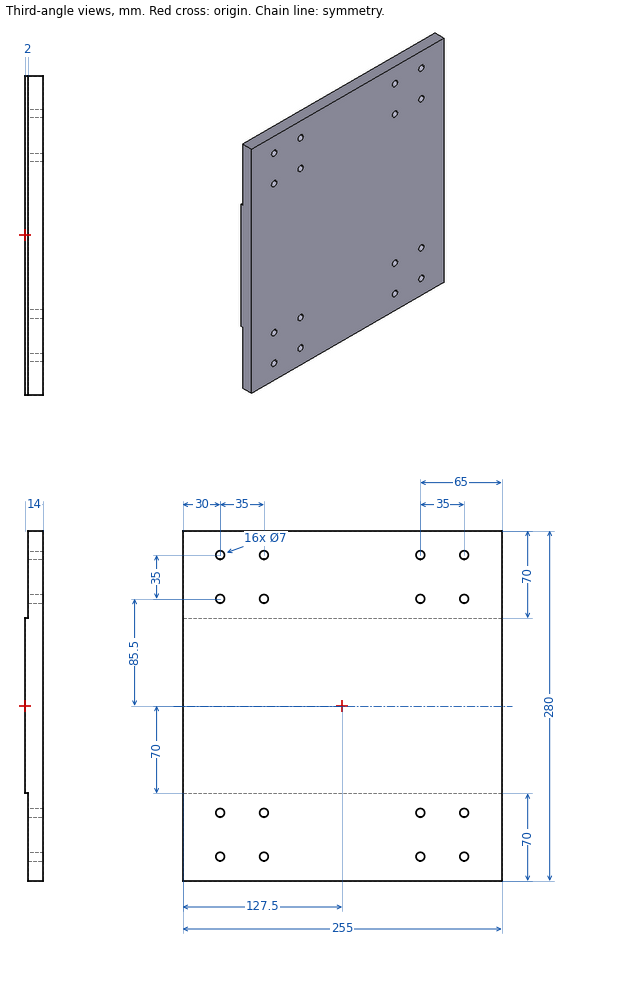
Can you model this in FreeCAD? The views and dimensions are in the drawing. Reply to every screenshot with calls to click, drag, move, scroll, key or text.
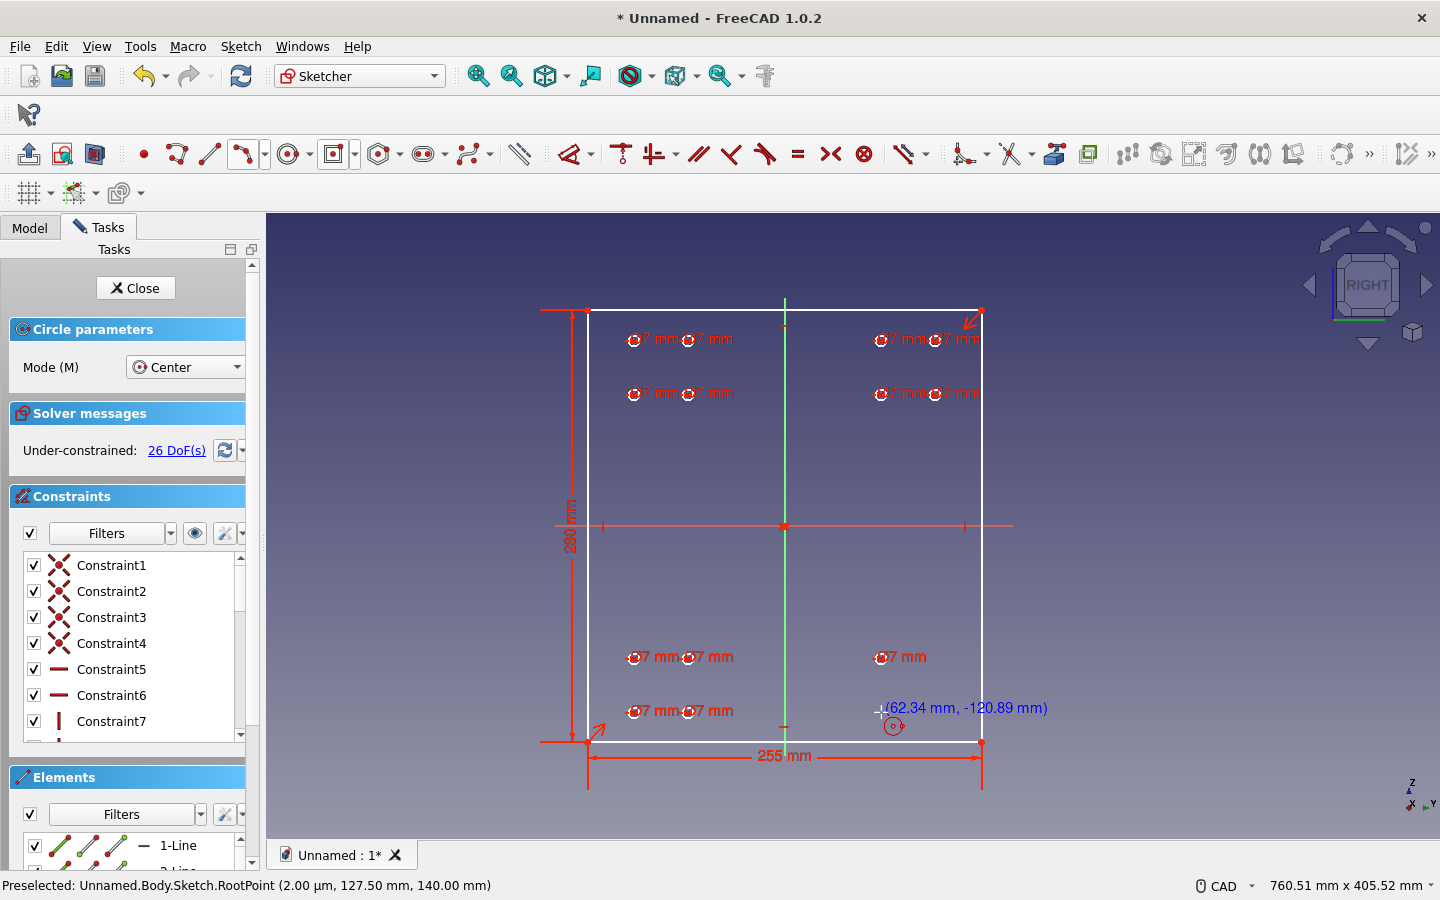
click(881, 712)
move(885, 709)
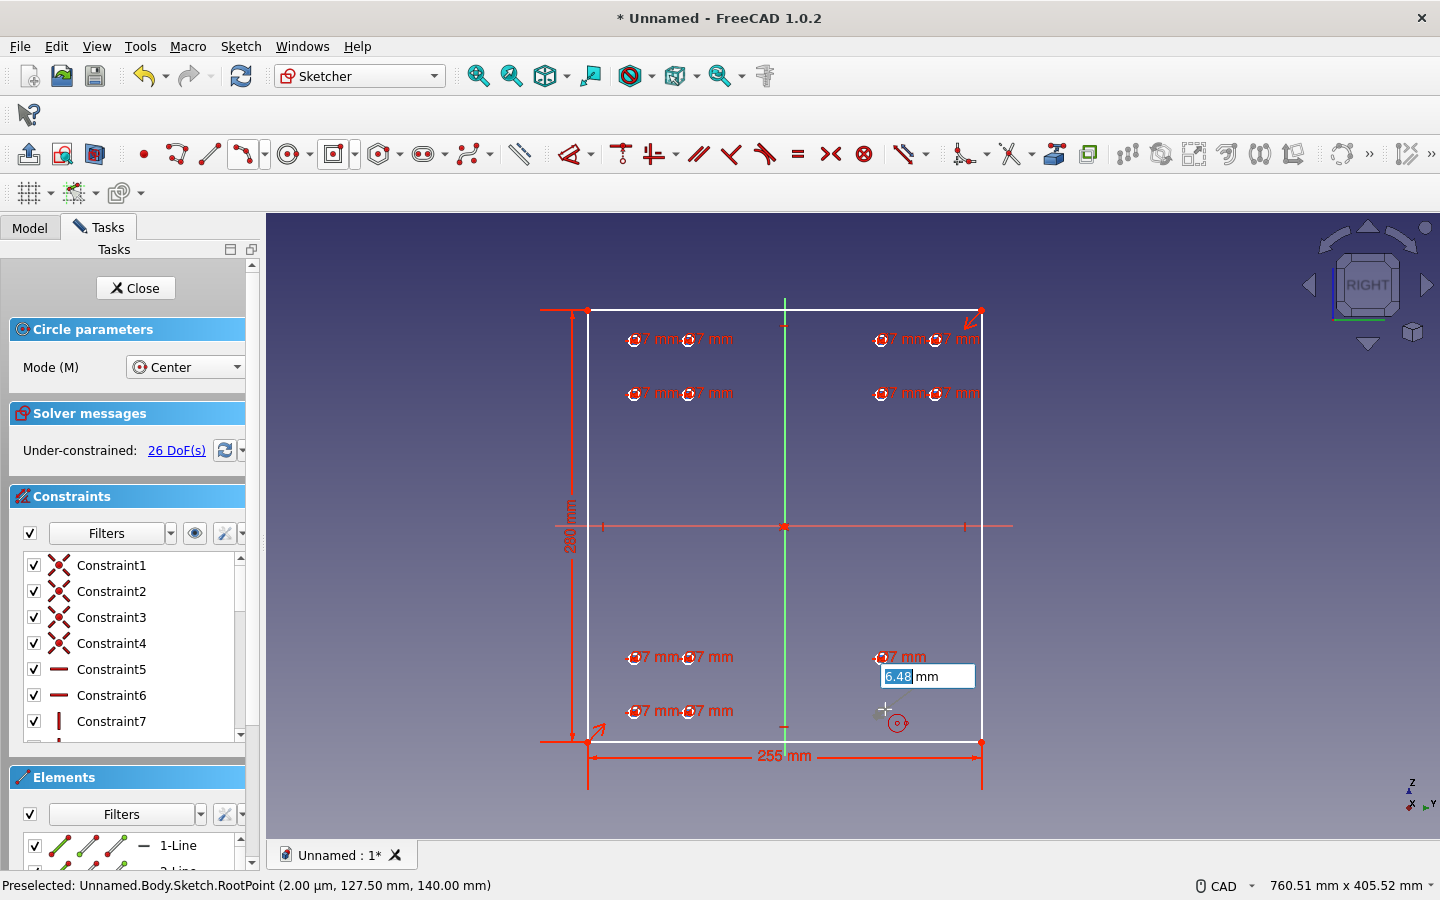
text(7)
key(Return)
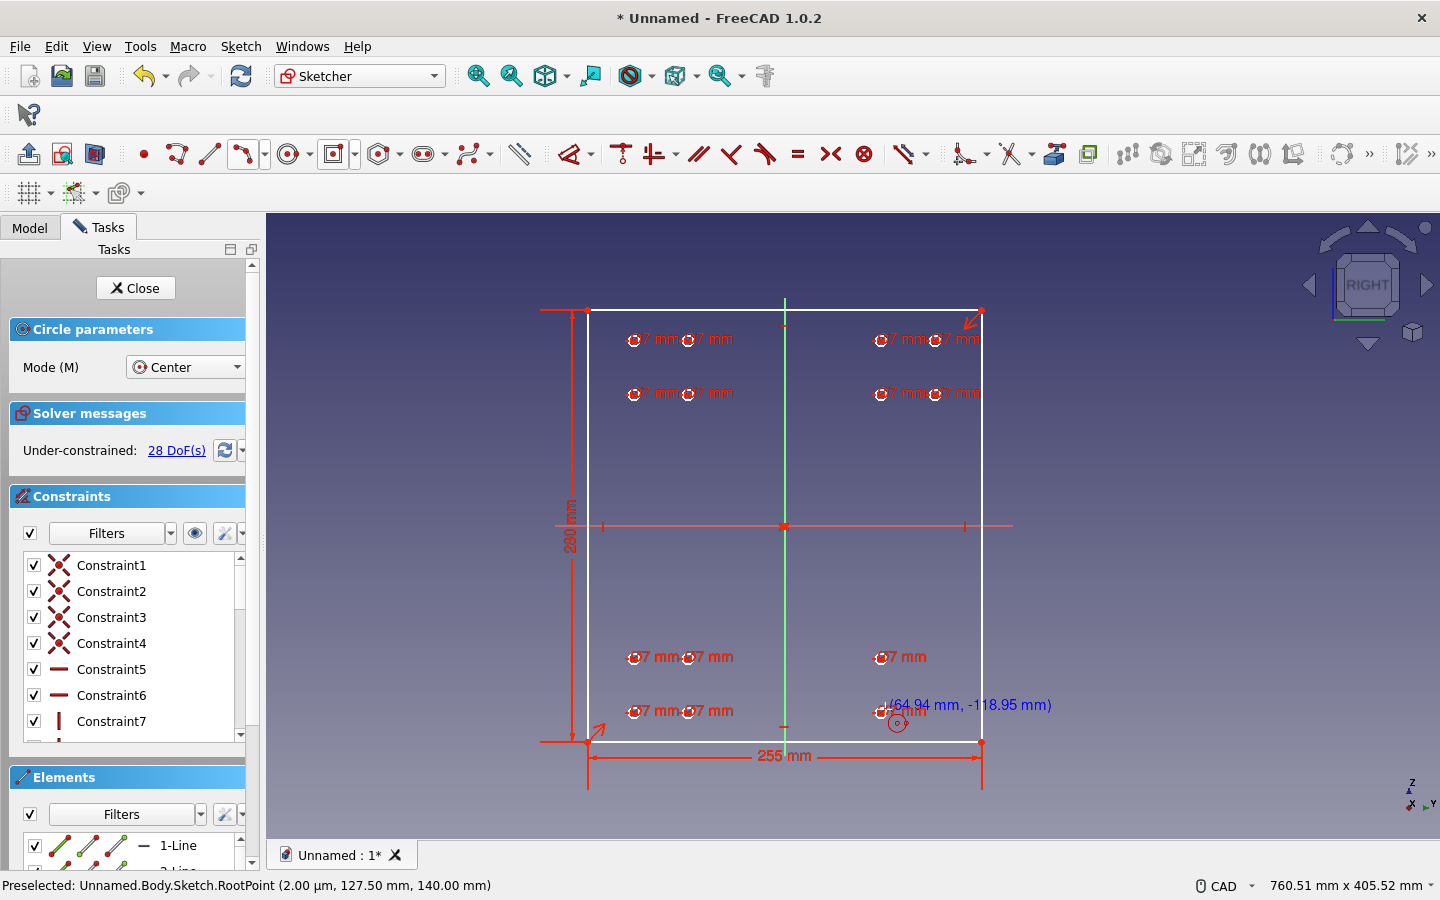
scroll(935, 658, up, 8)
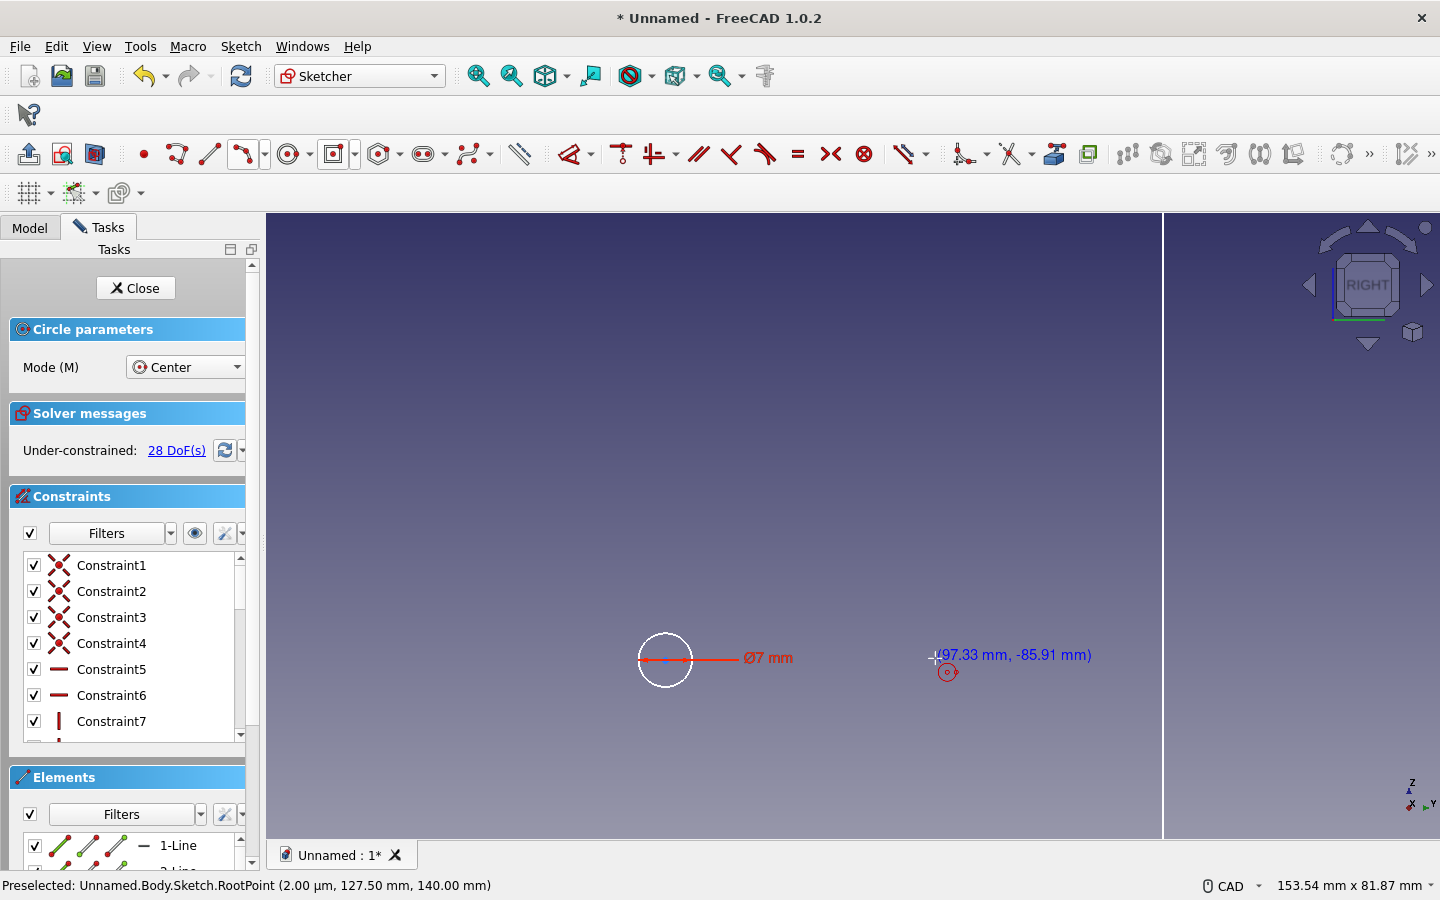
scroll(935, 658, down, 8)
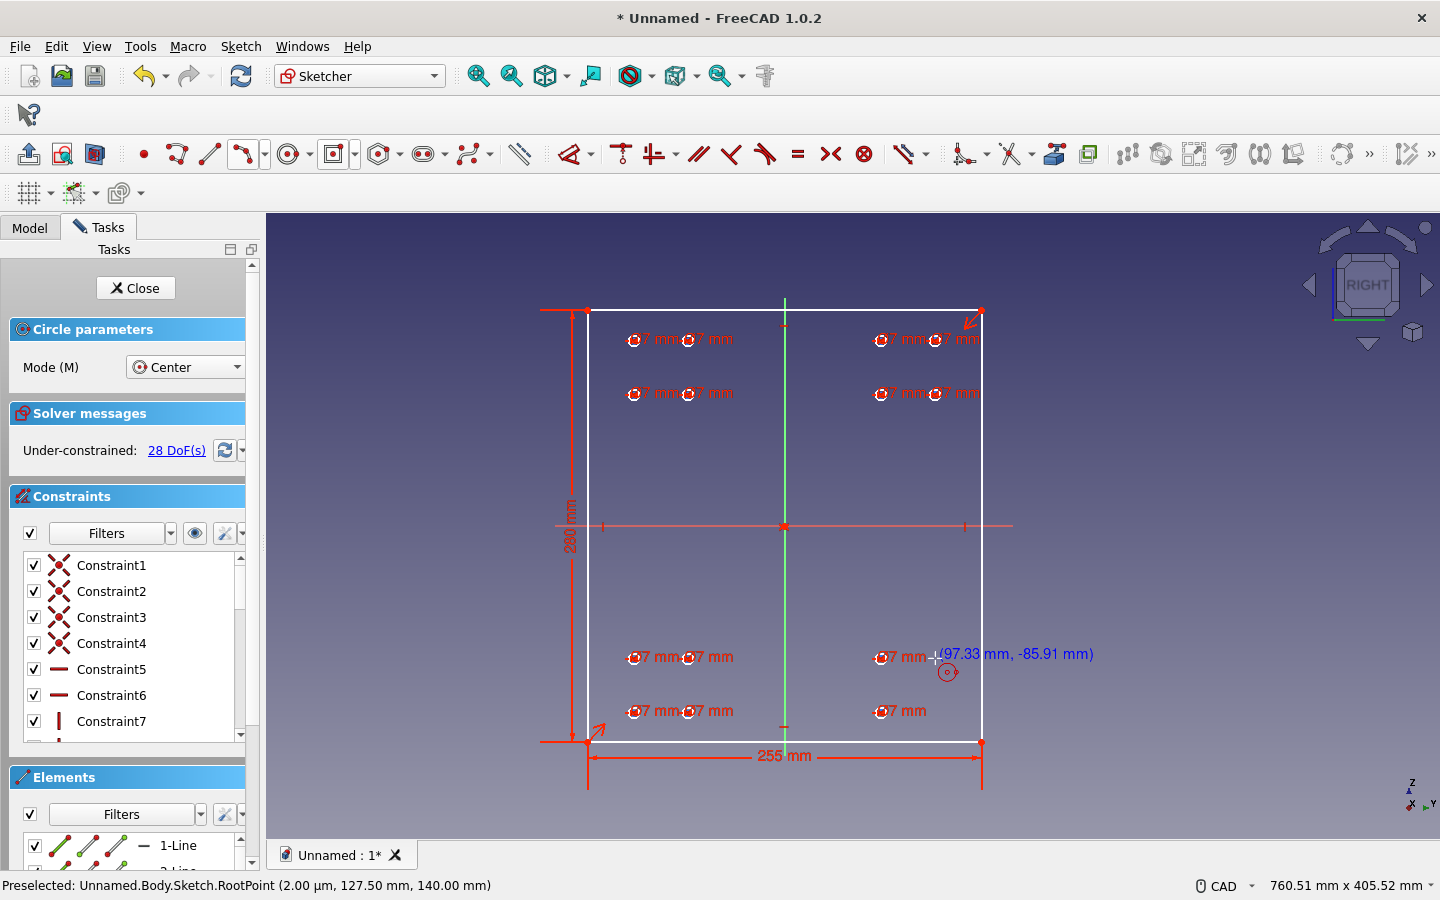
click(935, 658)
move(939, 655)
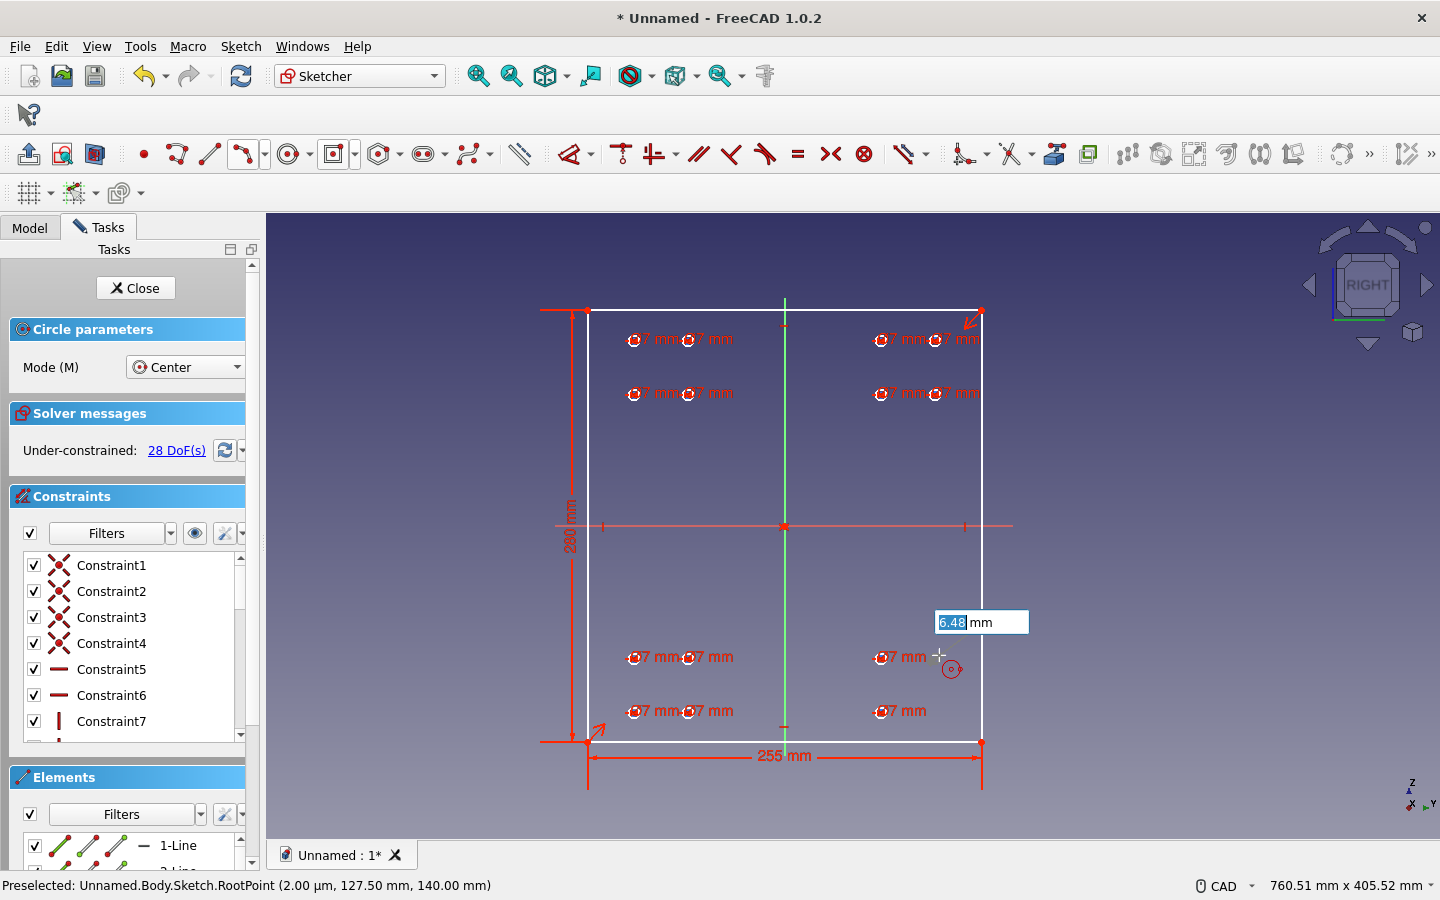
text(7)
key(Return)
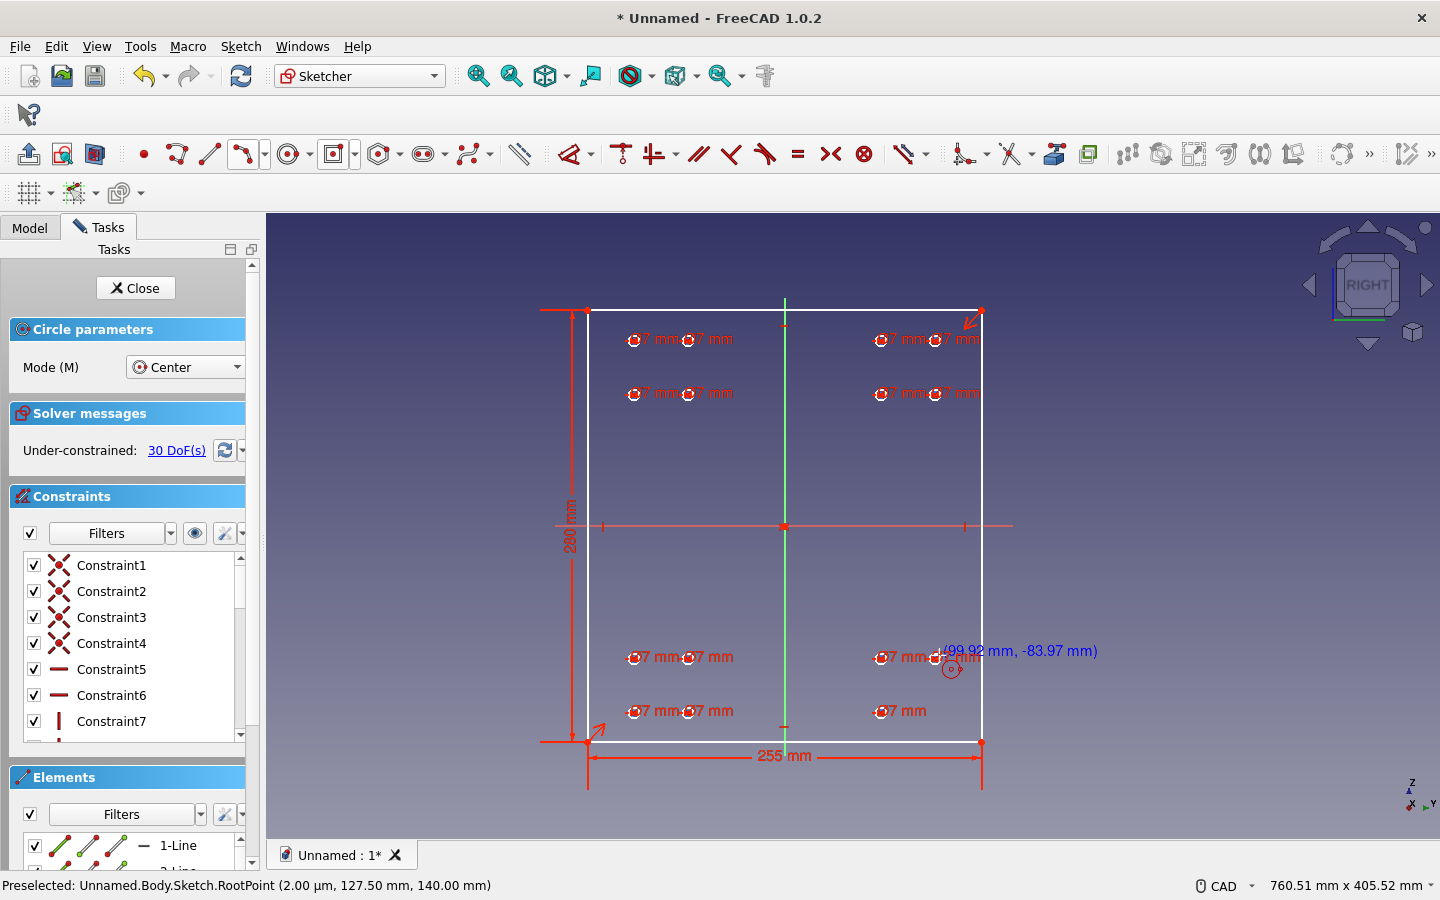
scroll(935, 712, up, 8)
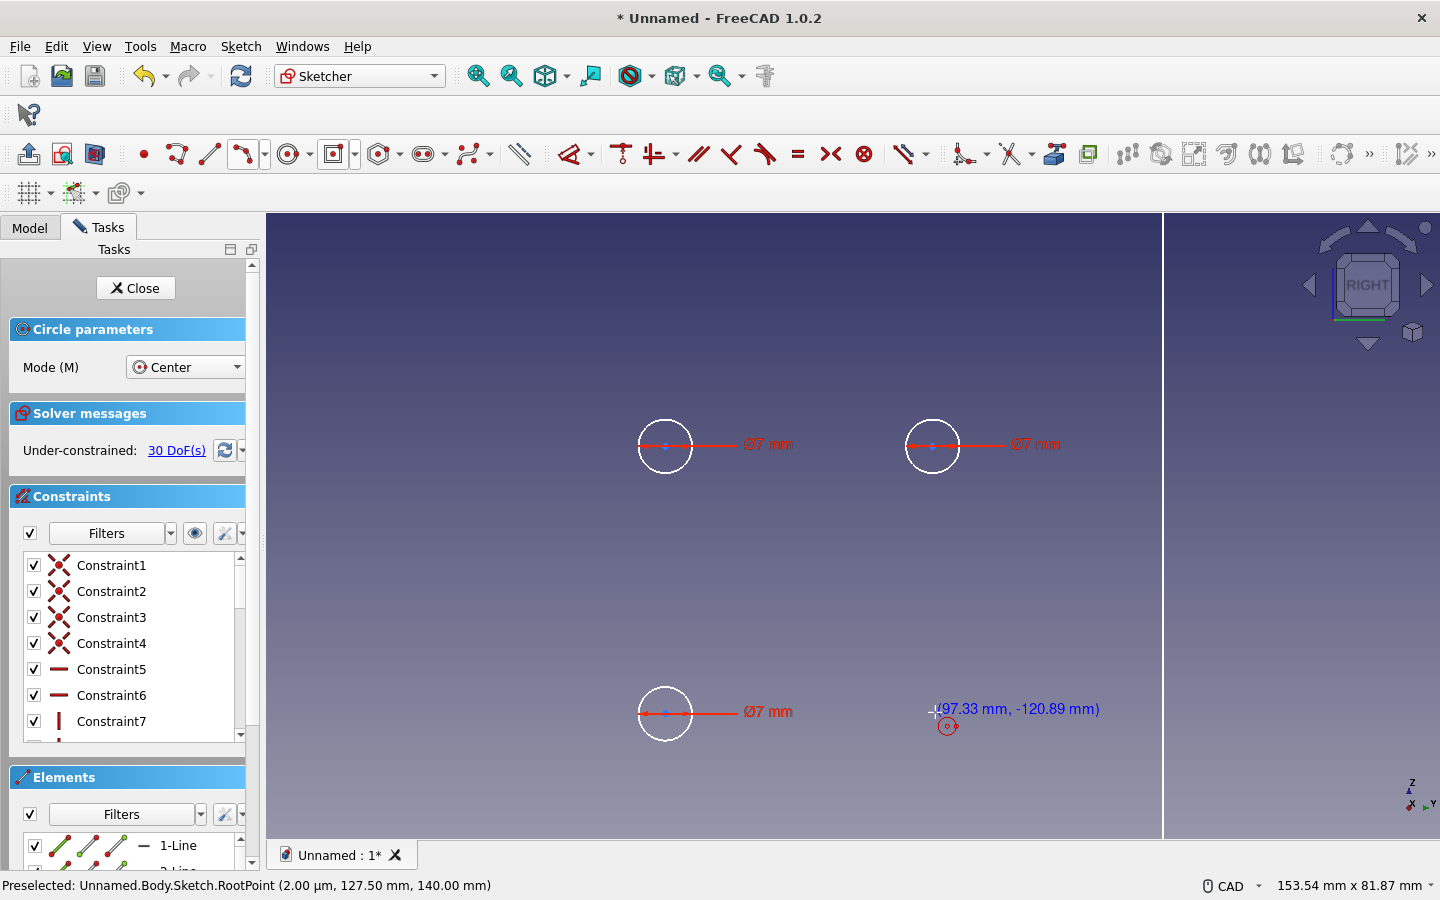
scroll(935, 712, down, 8)